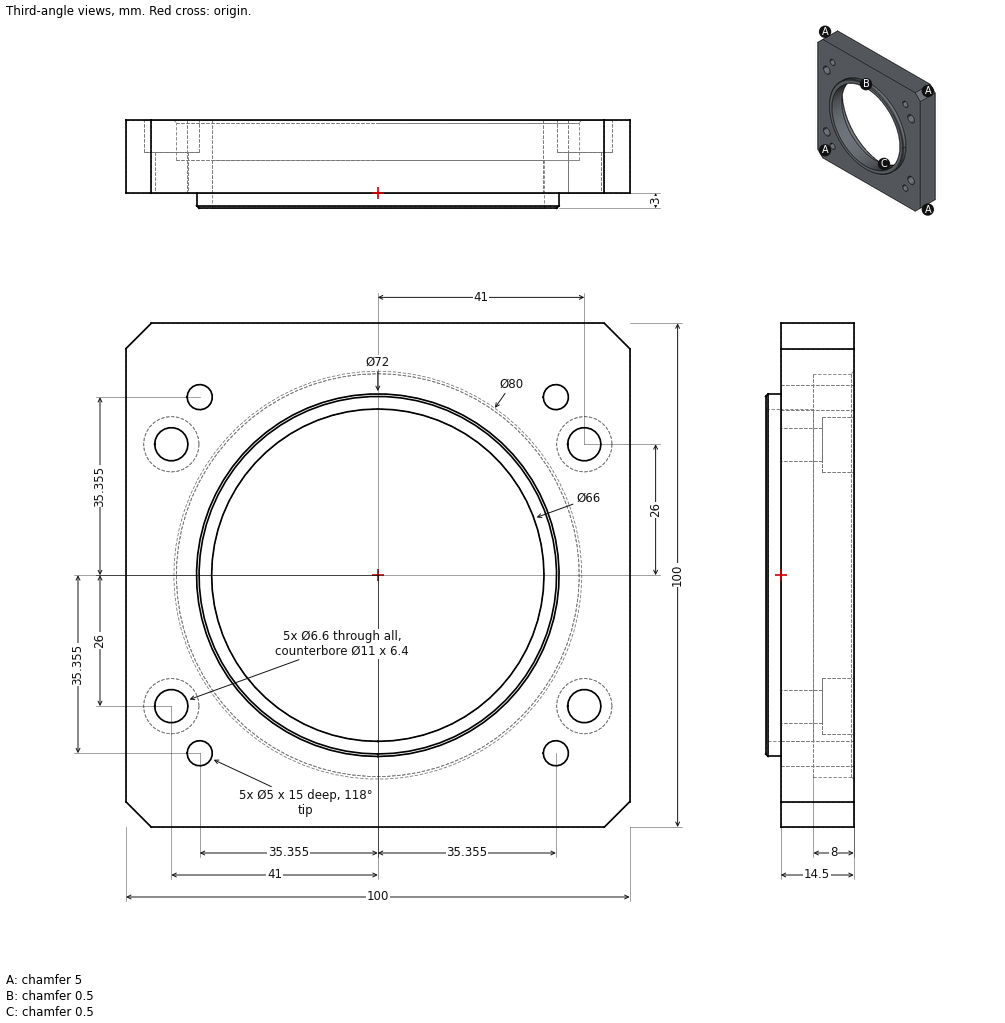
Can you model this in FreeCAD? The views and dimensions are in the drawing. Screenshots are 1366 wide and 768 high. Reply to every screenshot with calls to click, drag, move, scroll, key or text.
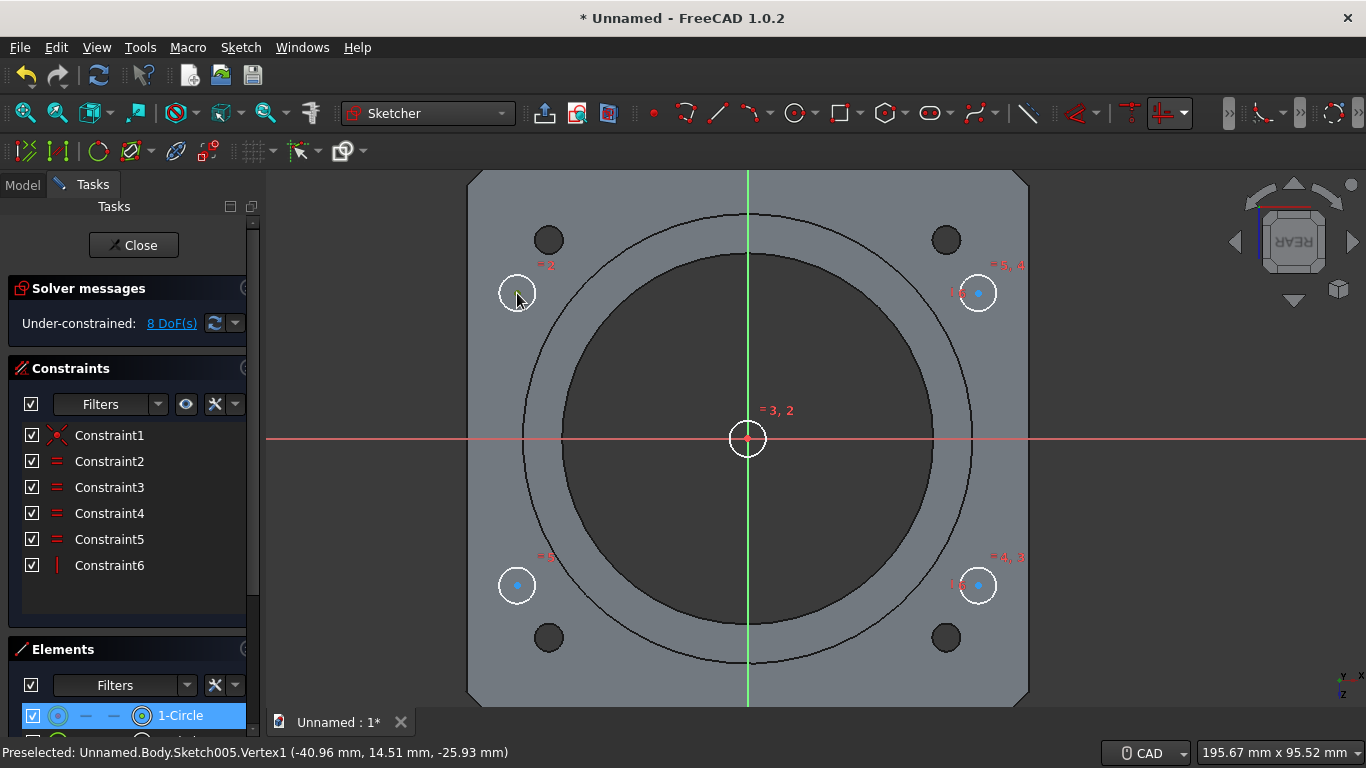
click(978, 293)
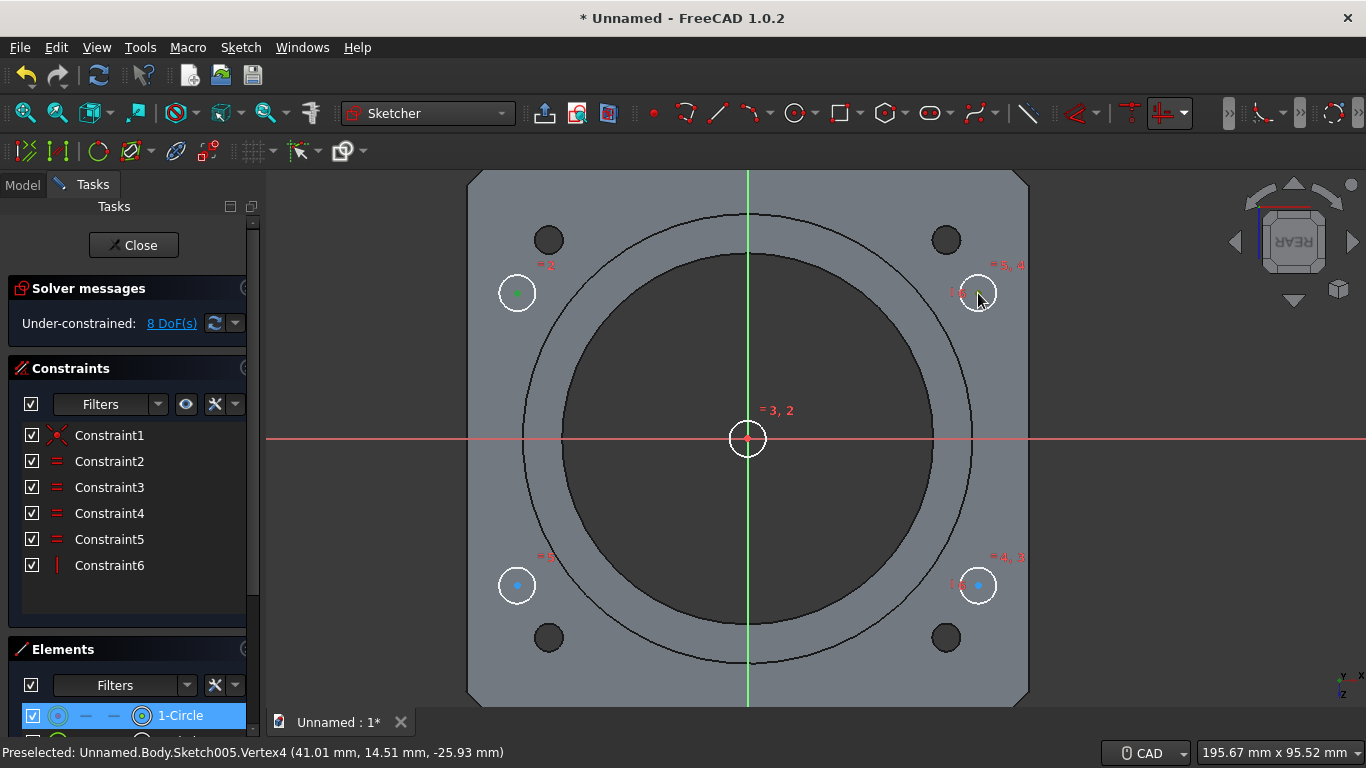
key(h)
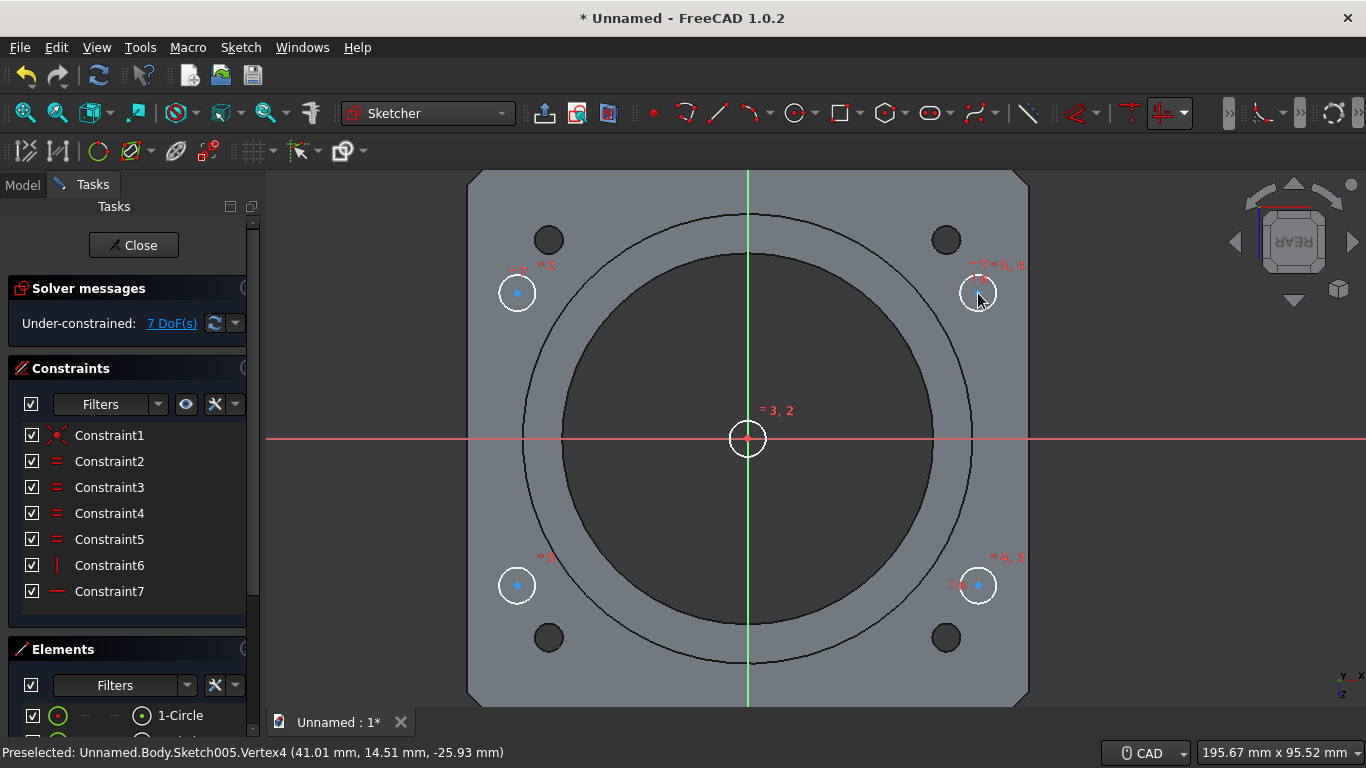
click(517, 293)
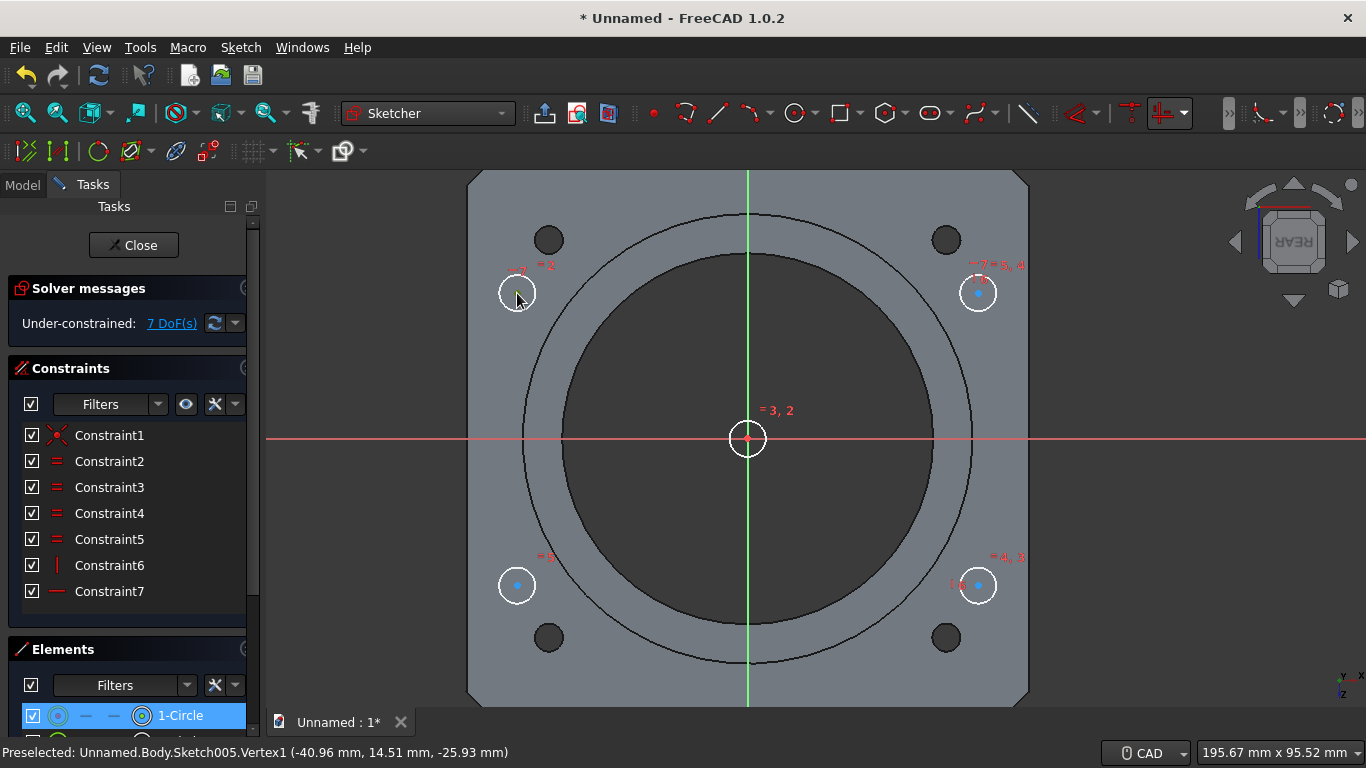
click(517, 586)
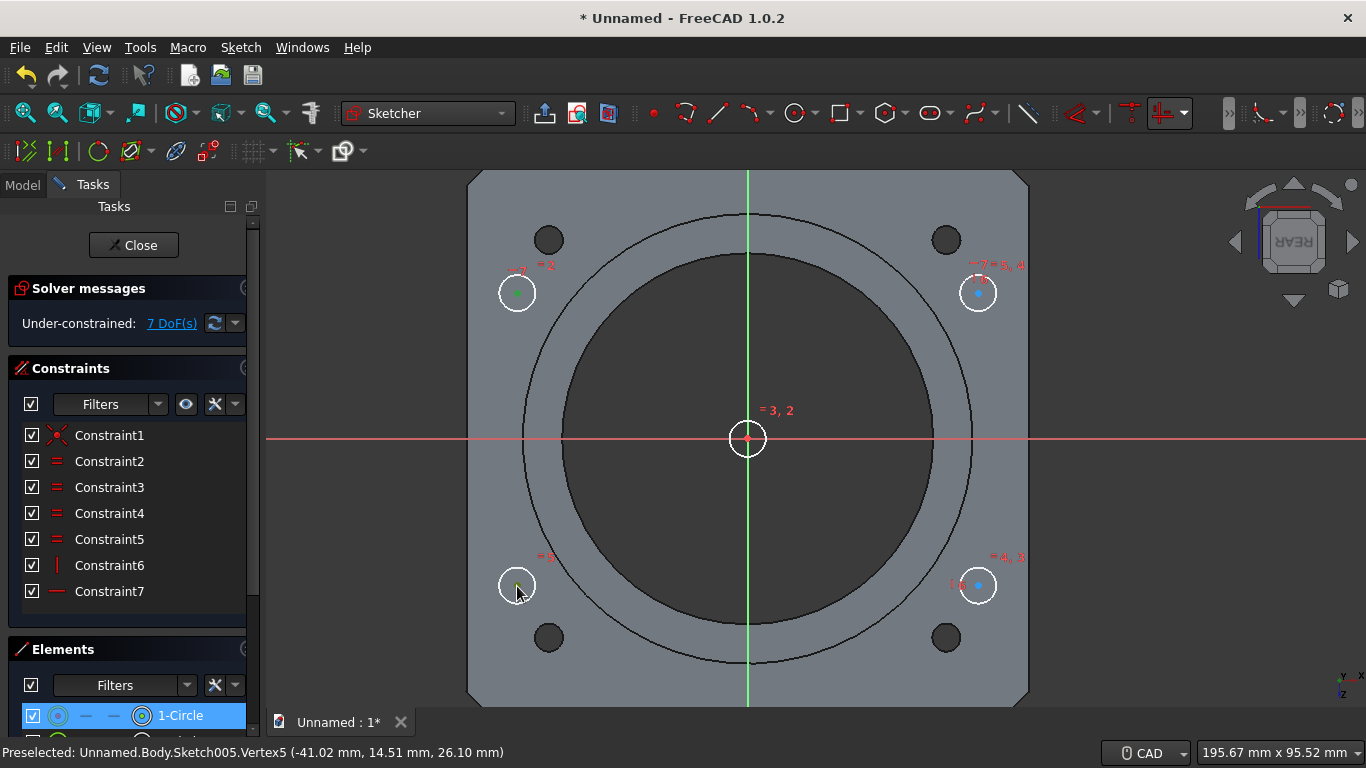
key(v)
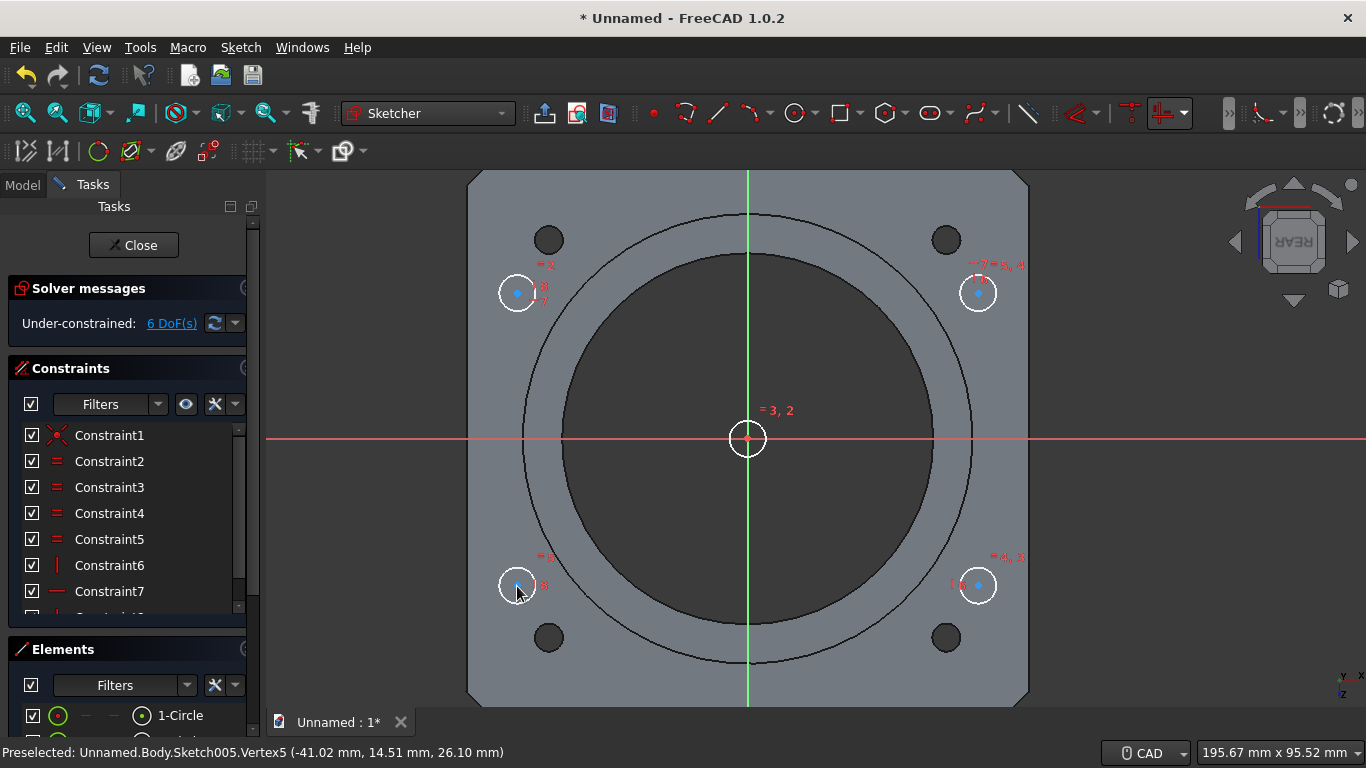
click(978, 586)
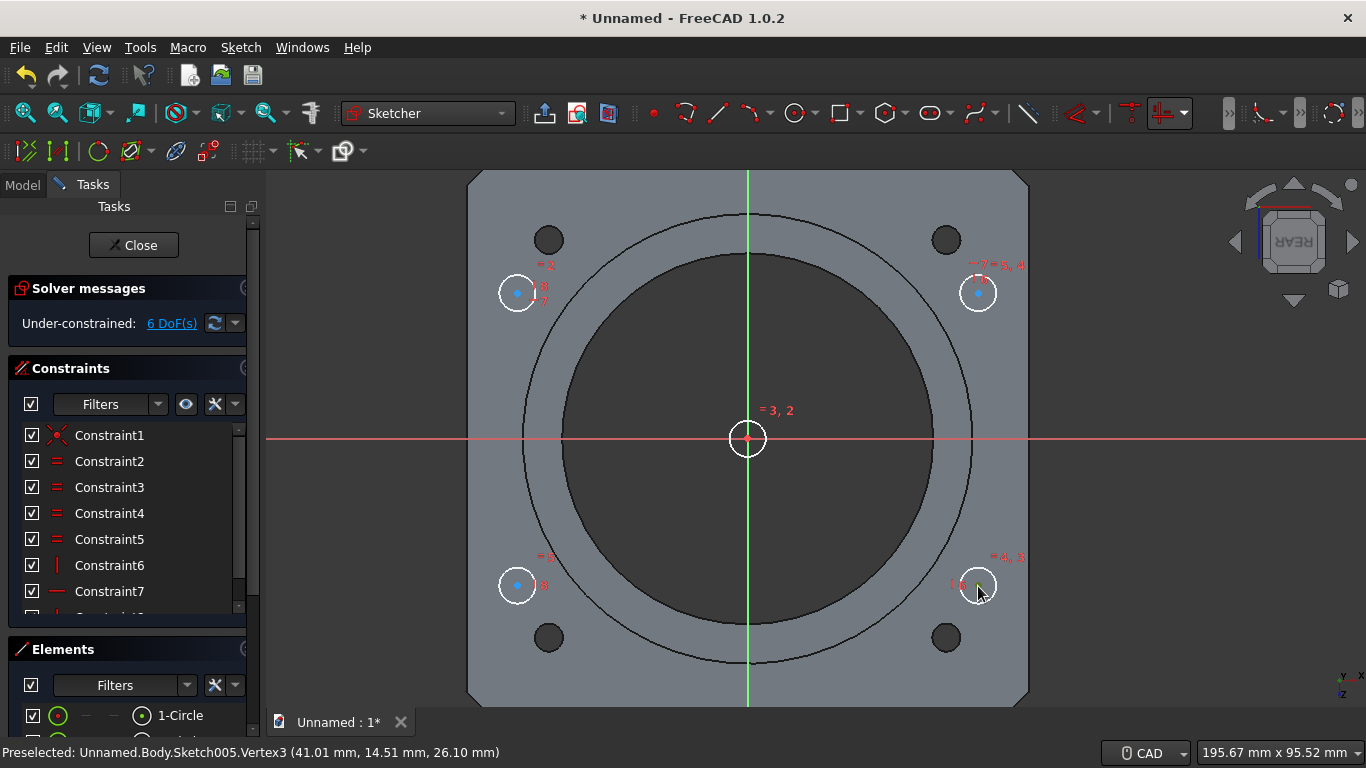
click(517, 586)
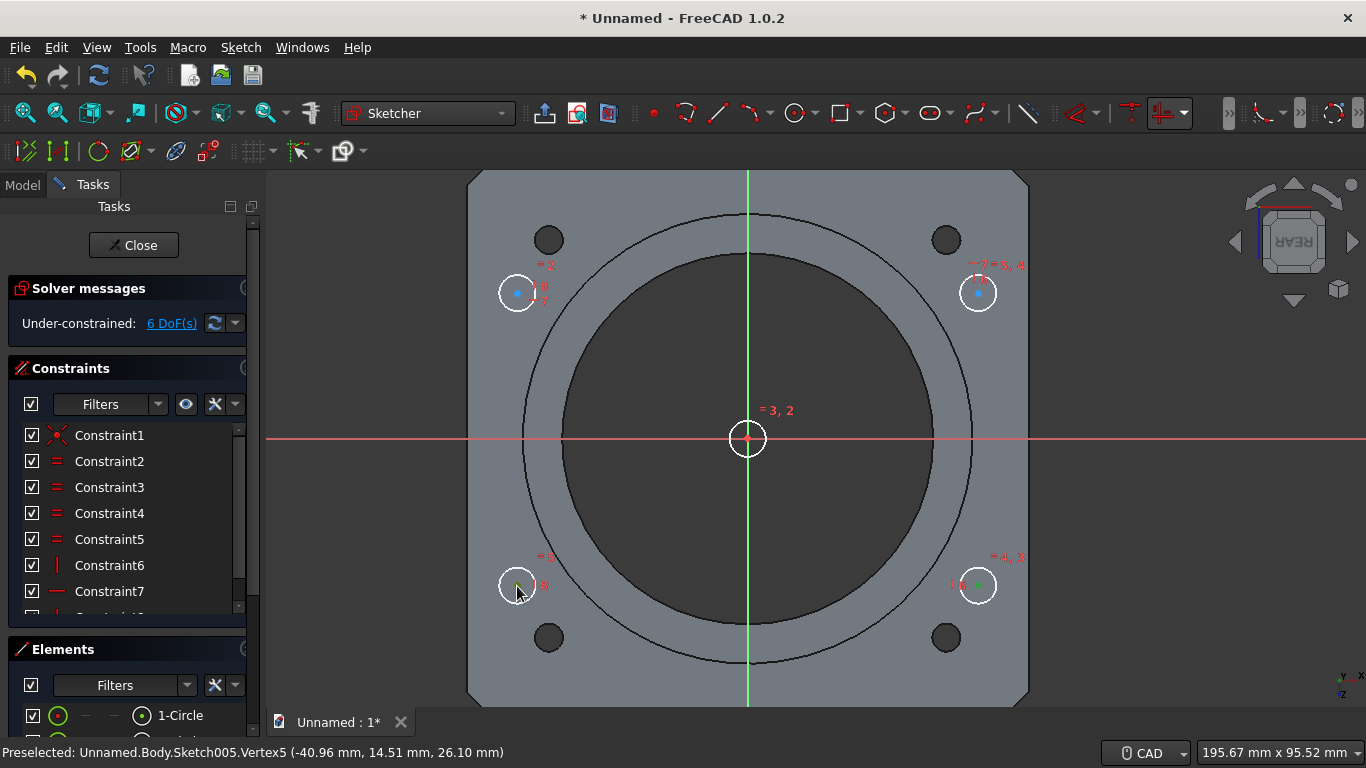
key(h)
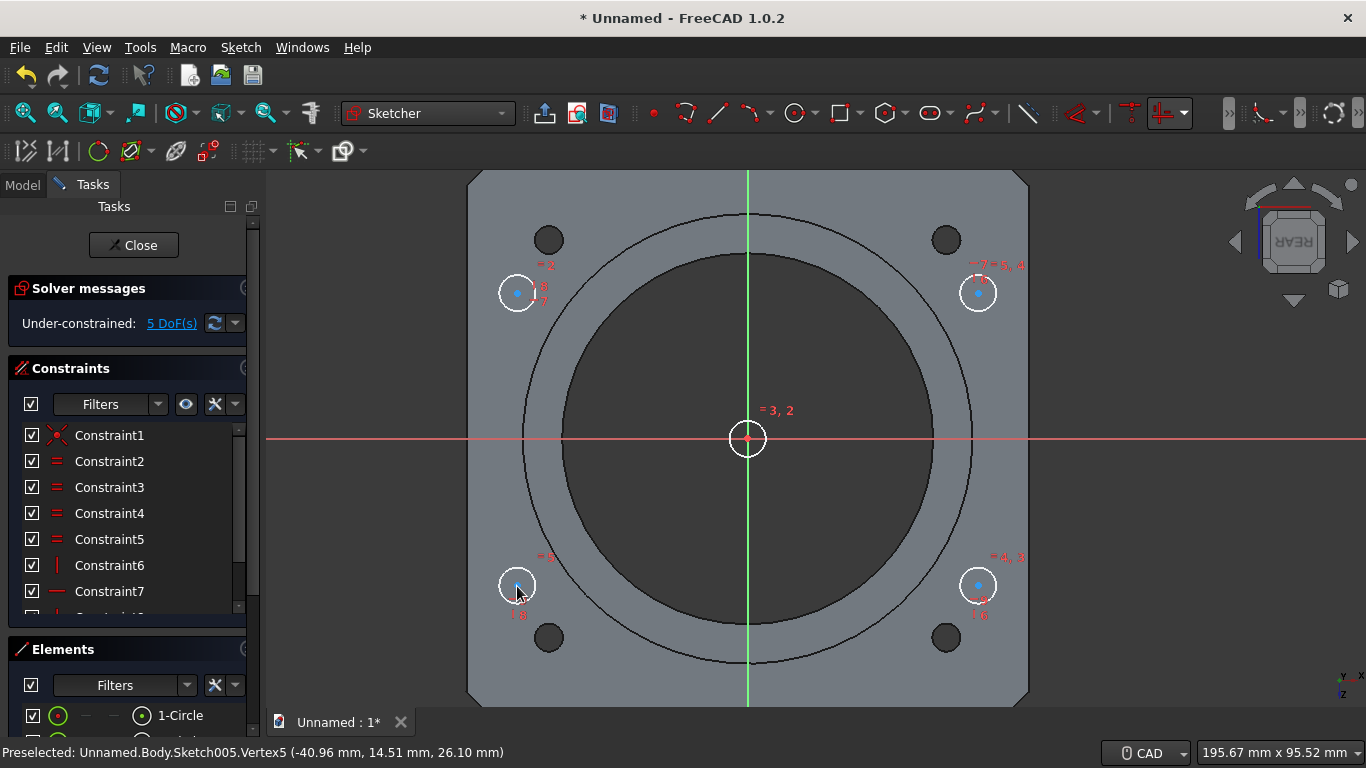
key(d)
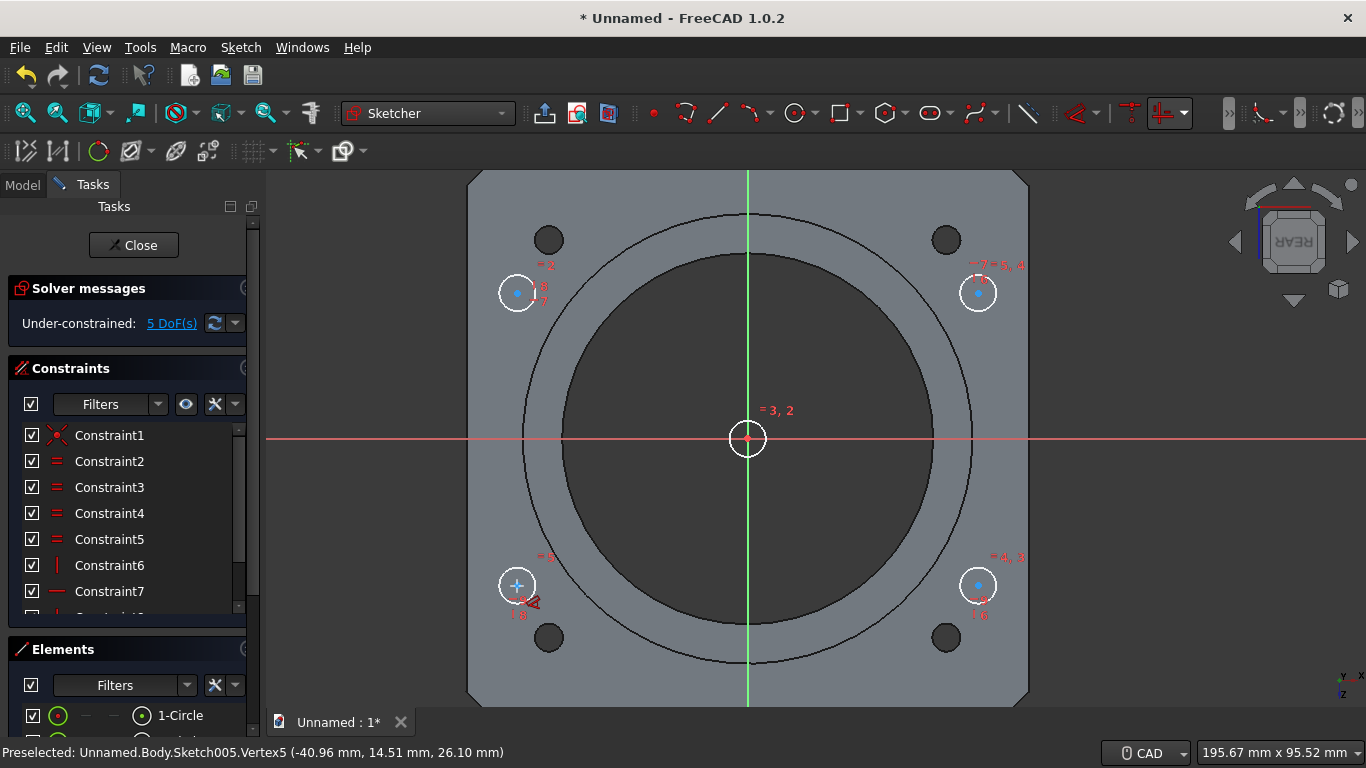
click(530, 280)
click(552, 257)